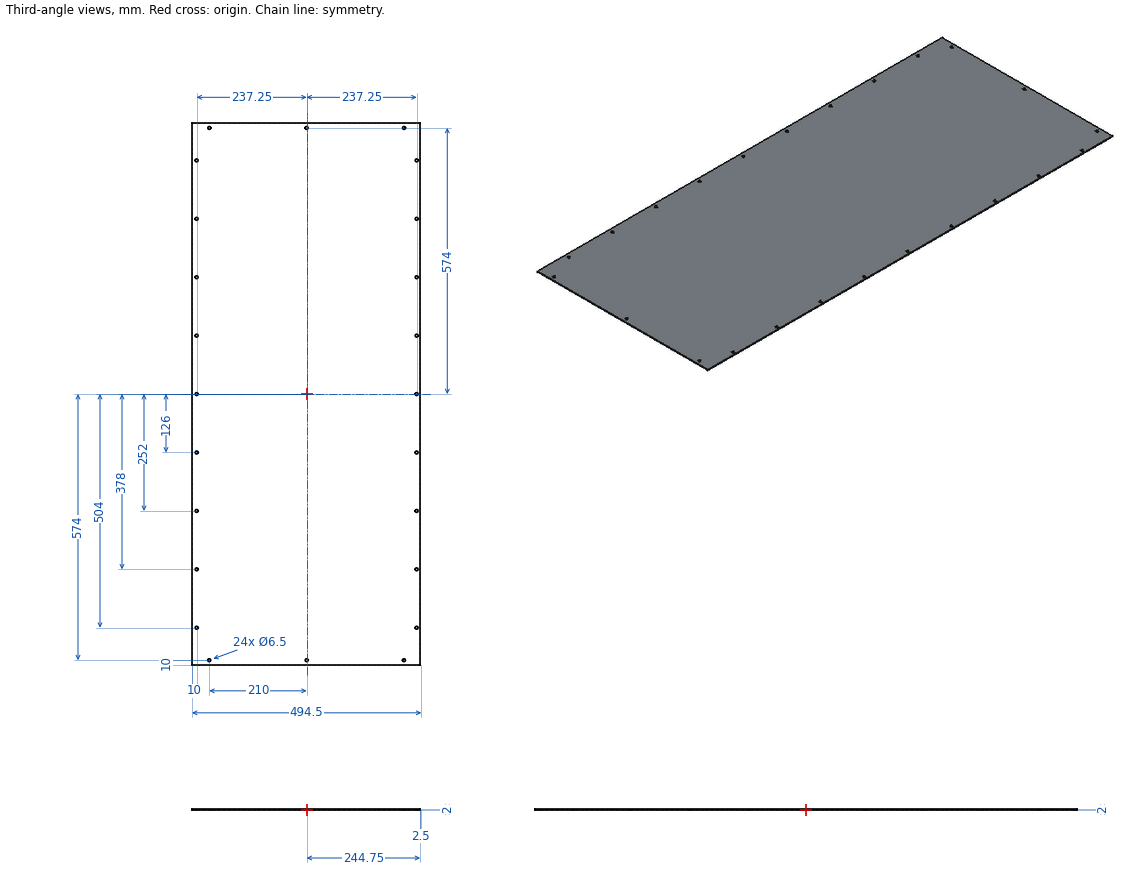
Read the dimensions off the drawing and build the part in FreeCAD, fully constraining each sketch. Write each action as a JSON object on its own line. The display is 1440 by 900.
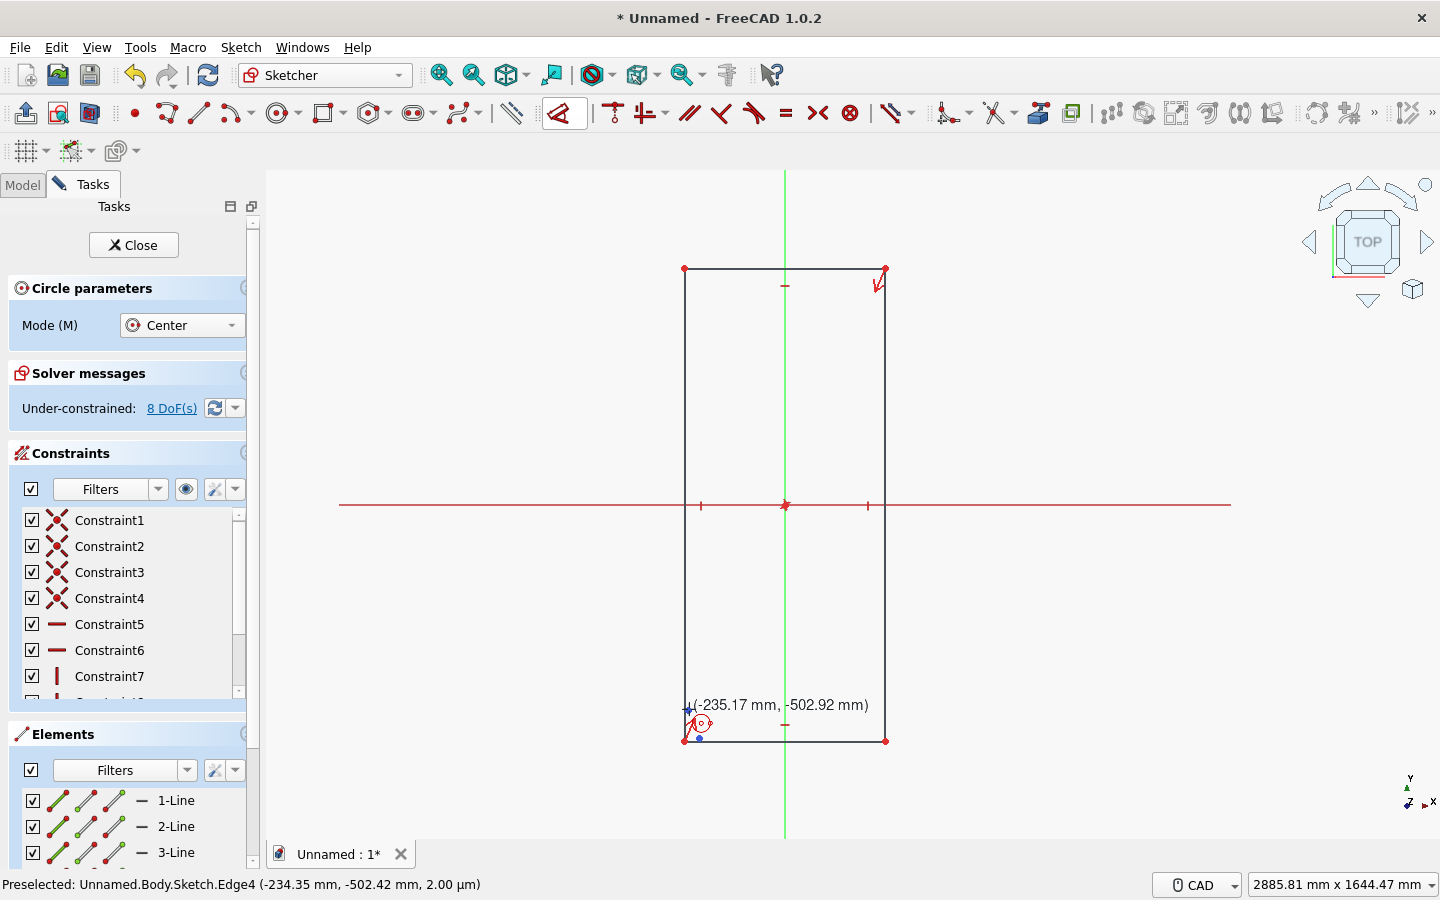
{"action": "scroll", "coordinate": [688, 659], "scroll_direction": "up", "scroll_amount": 15}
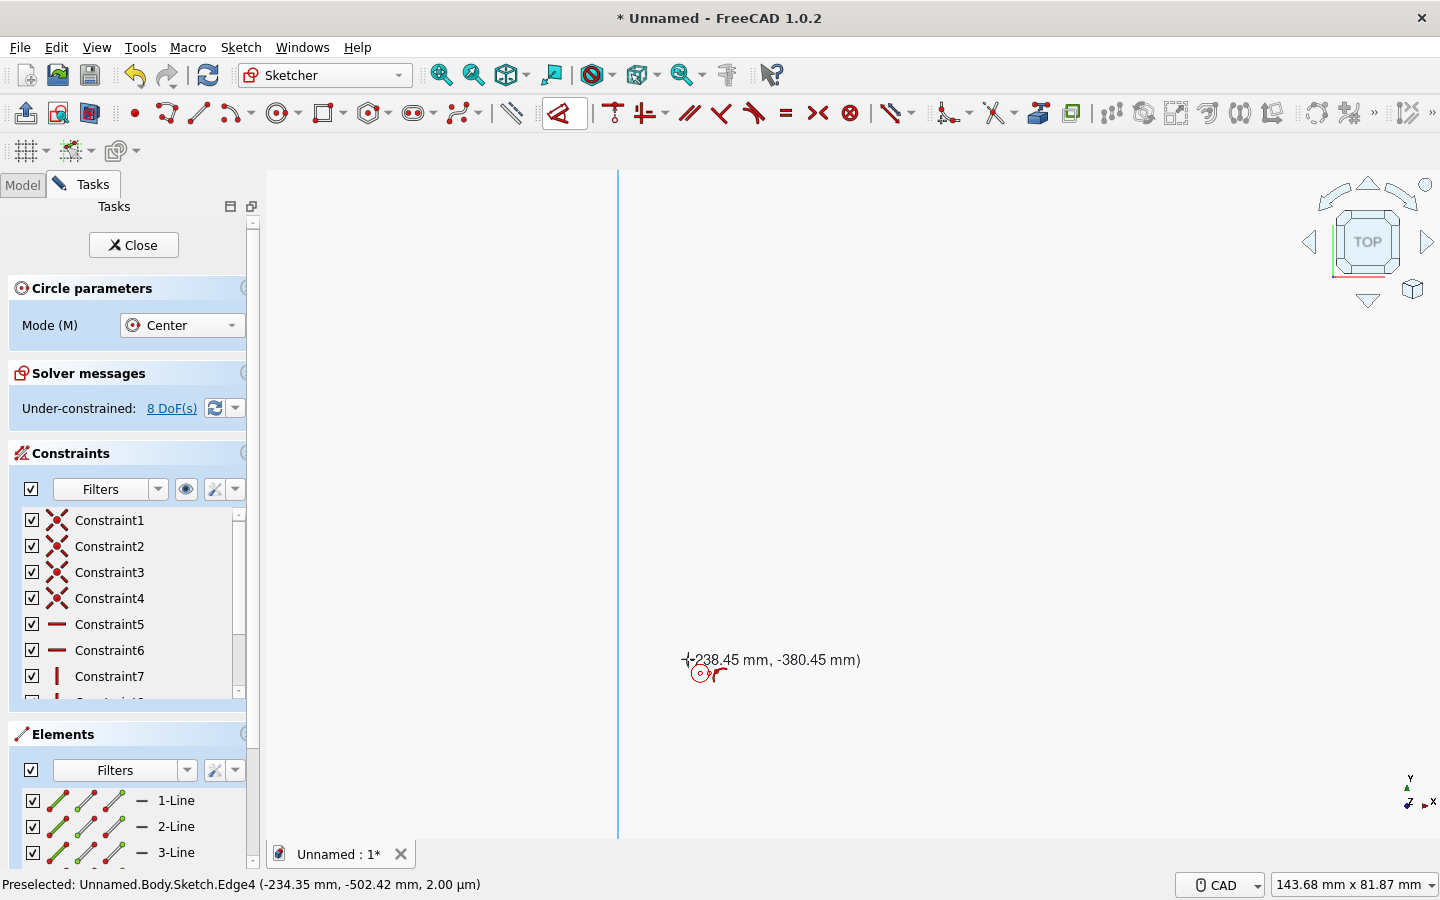
{"action": "scroll", "coordinate": [688, 659], "scroll_direction": "down", "scroll_amount": 15}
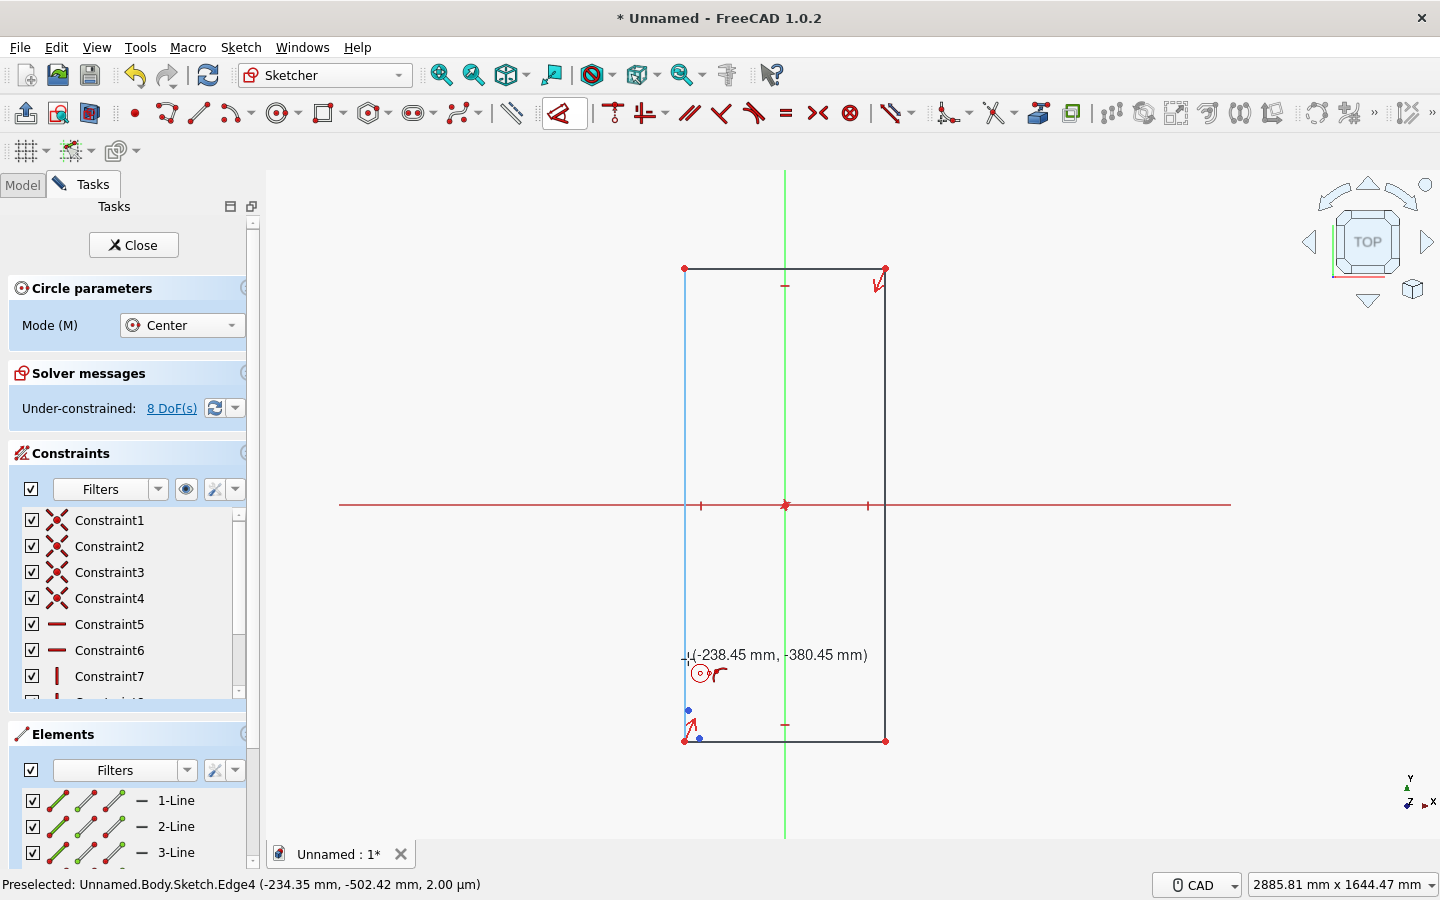
{"action": "scroll", "coordinate": [688, 659], "scroll_direction": "up", "scroll_amount": 7}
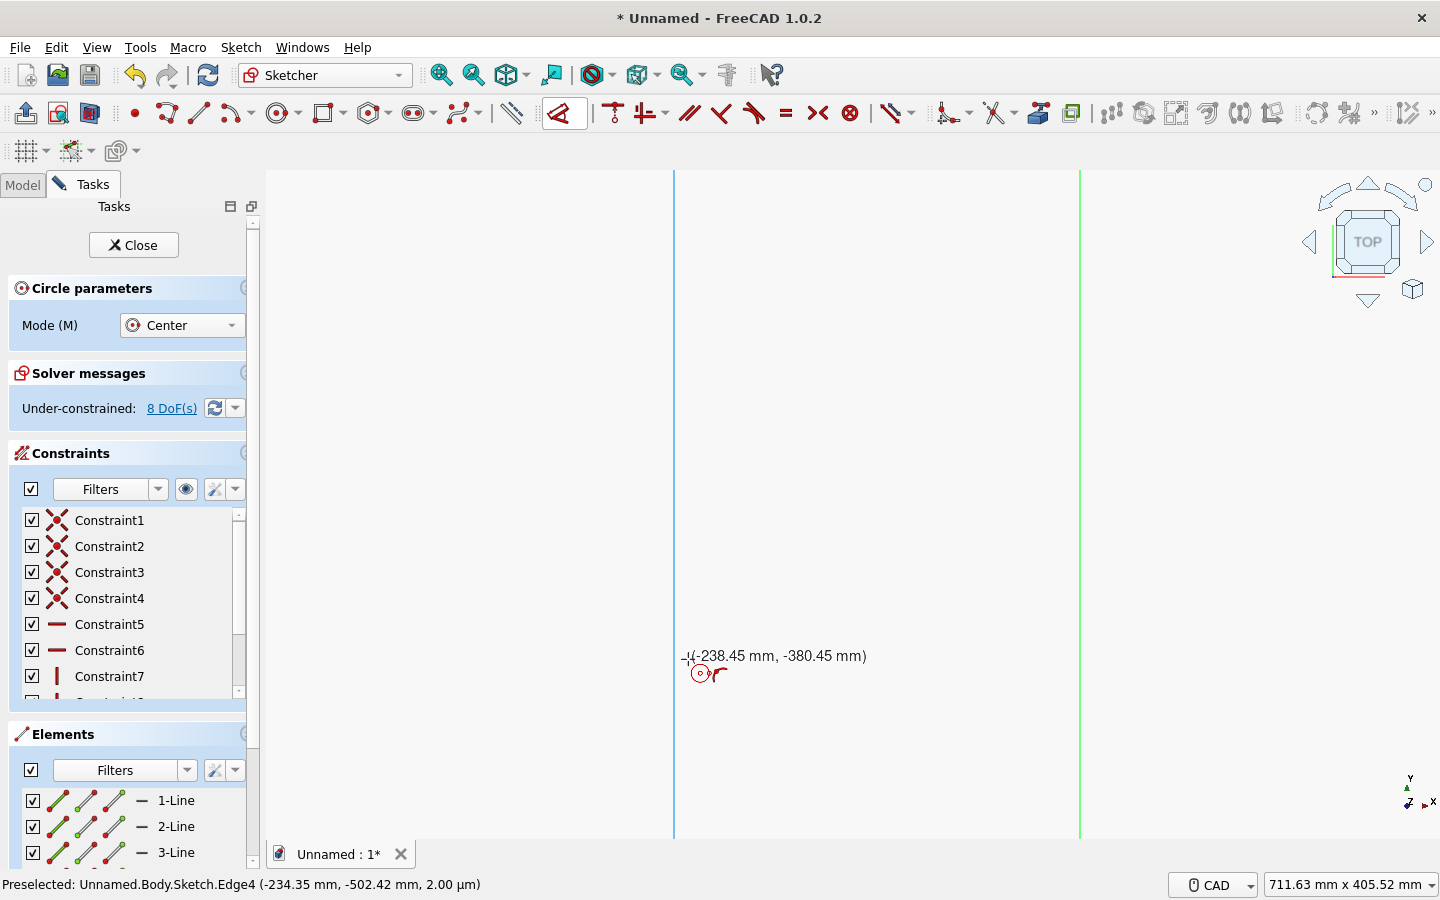
{"action": "left_click", "coordinate": [689, 657]}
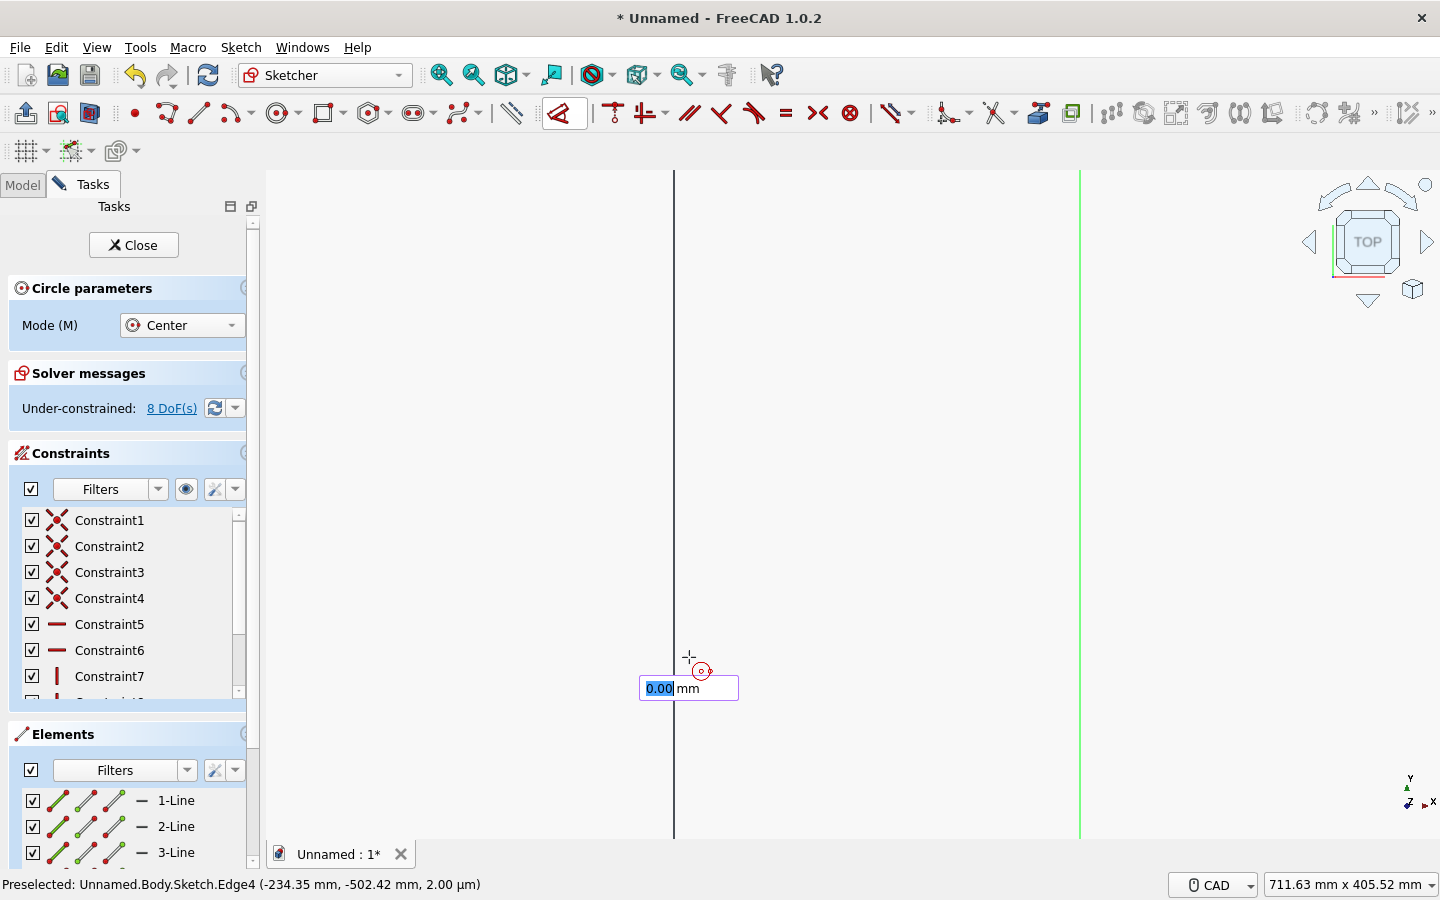
{"action": "scroll", "coordinate": [693, 653], "scroll_direction": "up", "scroll_amount": 6}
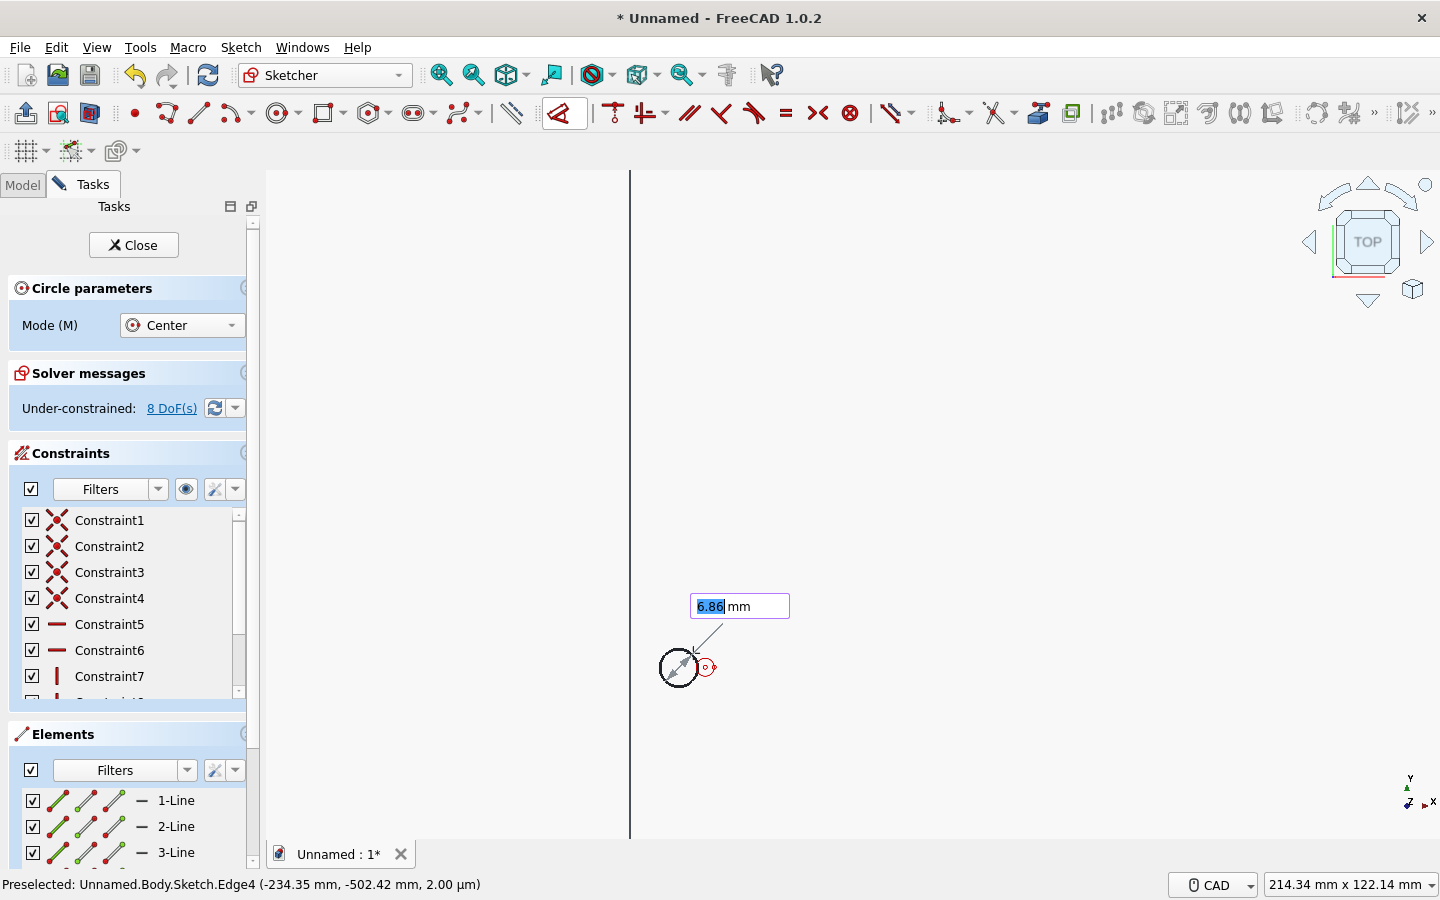
{"action": "left_click", "coordinate": [691, 651]}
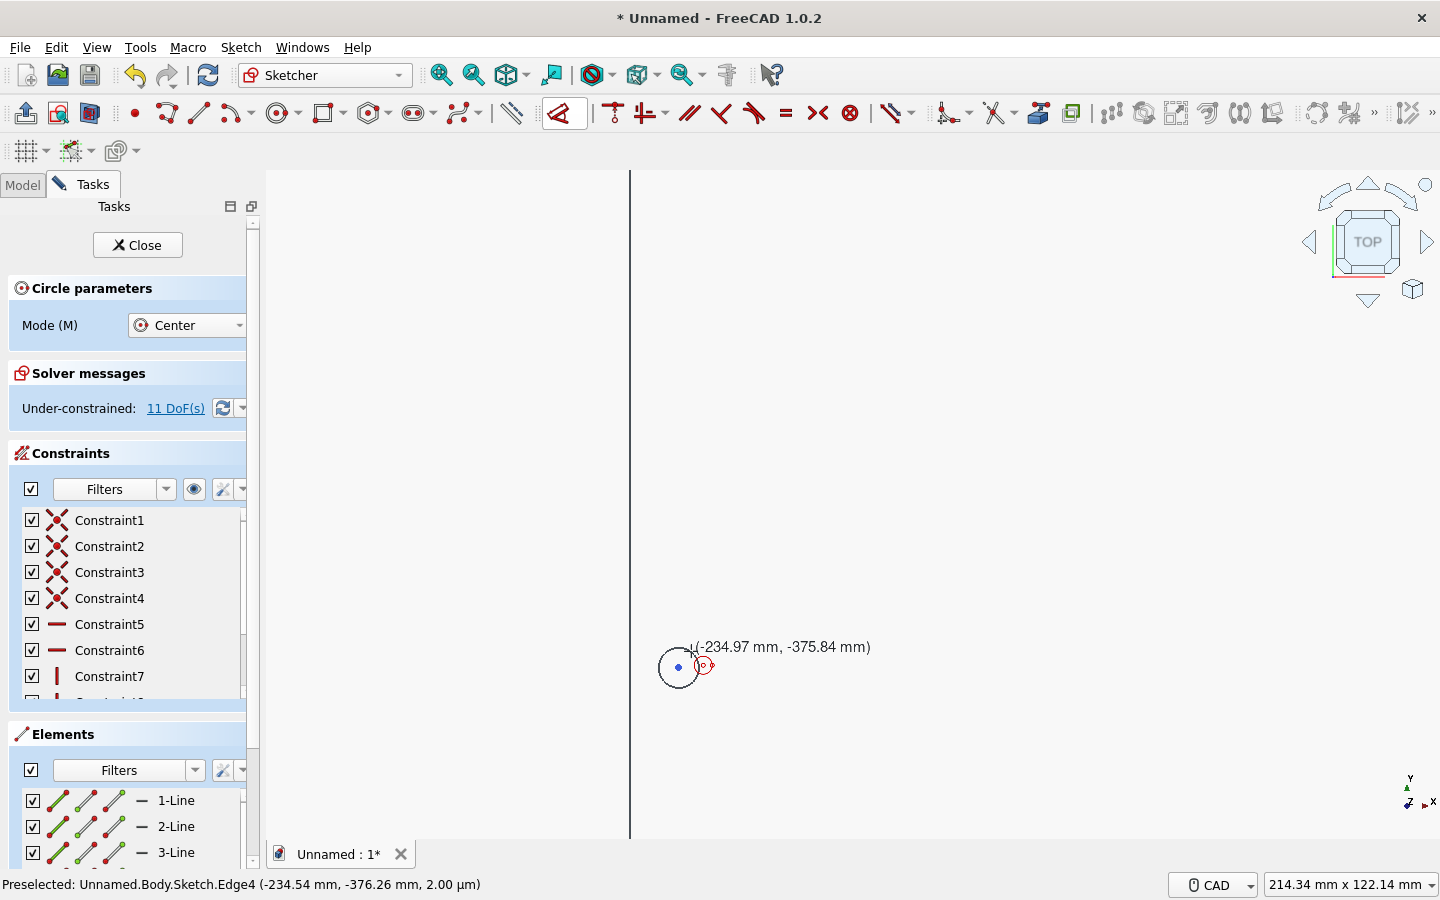
{"action": "scroll", "coordinate": [689, 658], "scroll_direction": "down", "scroll_amount": 13}